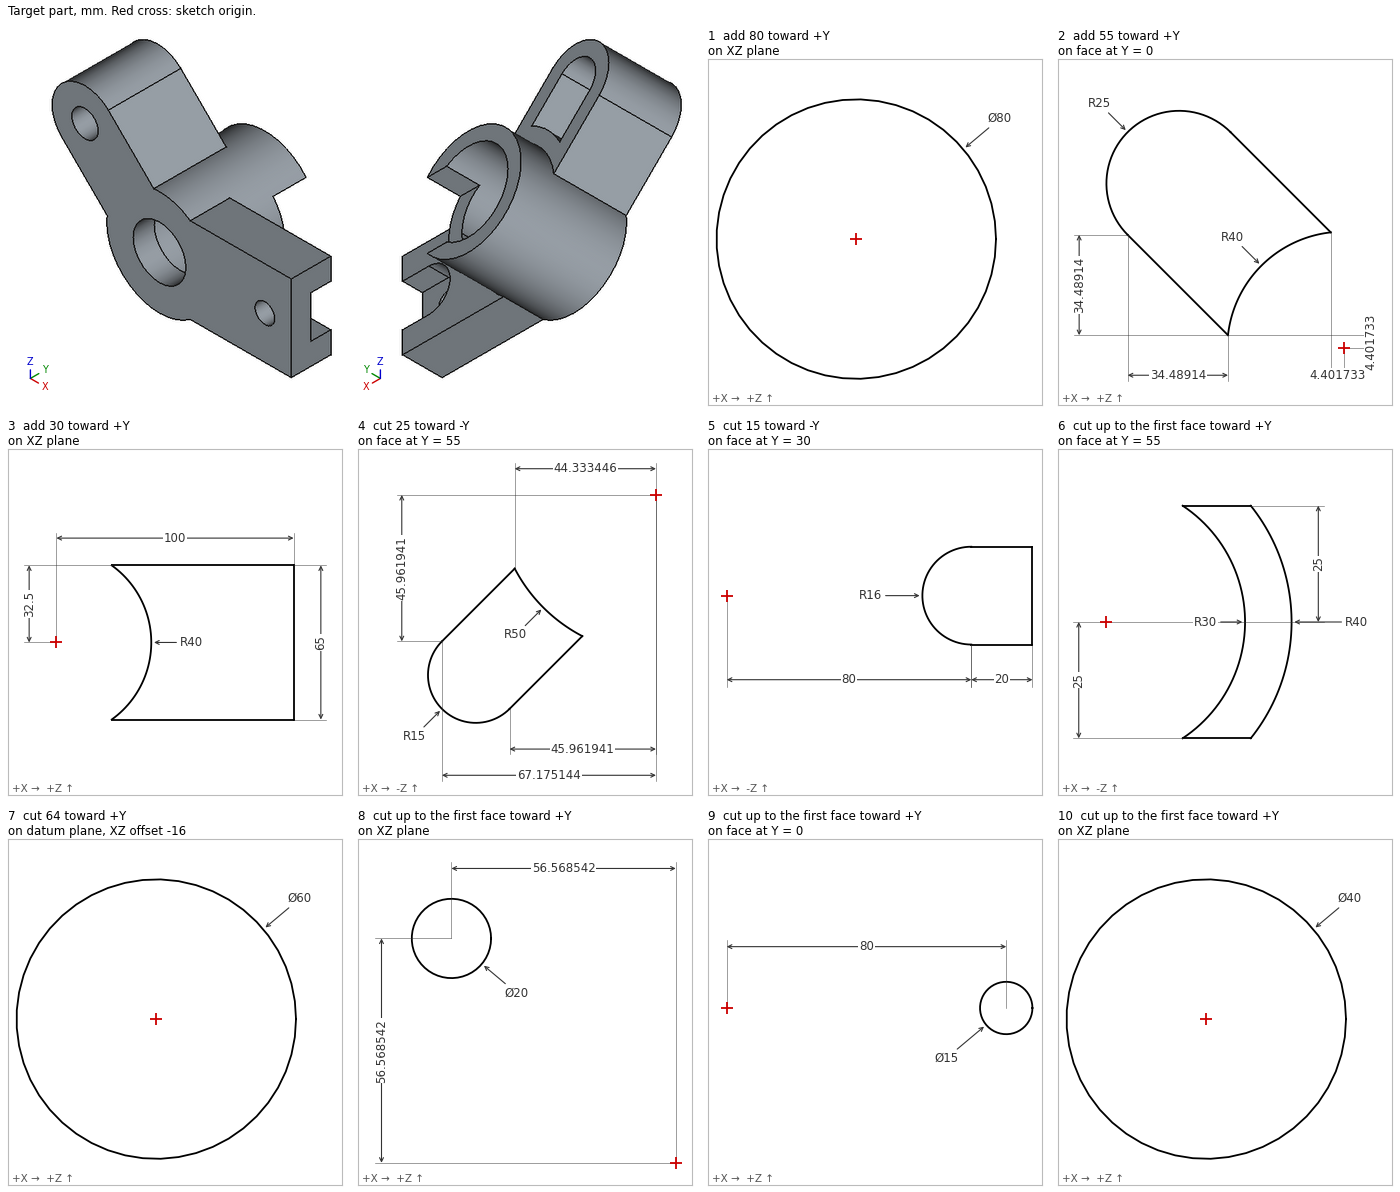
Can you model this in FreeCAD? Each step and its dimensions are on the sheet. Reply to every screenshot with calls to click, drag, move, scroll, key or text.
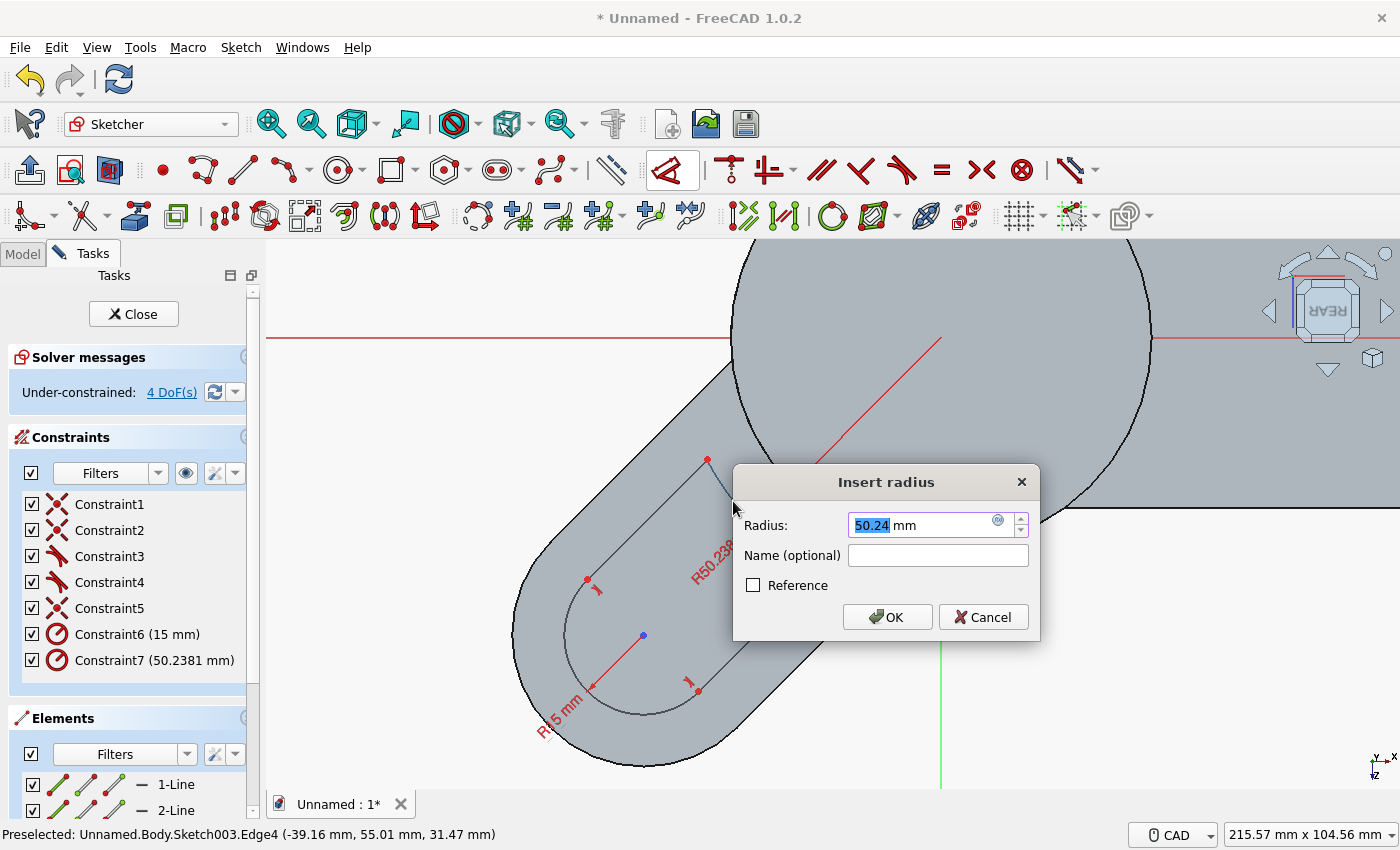
text(50)
key(Return)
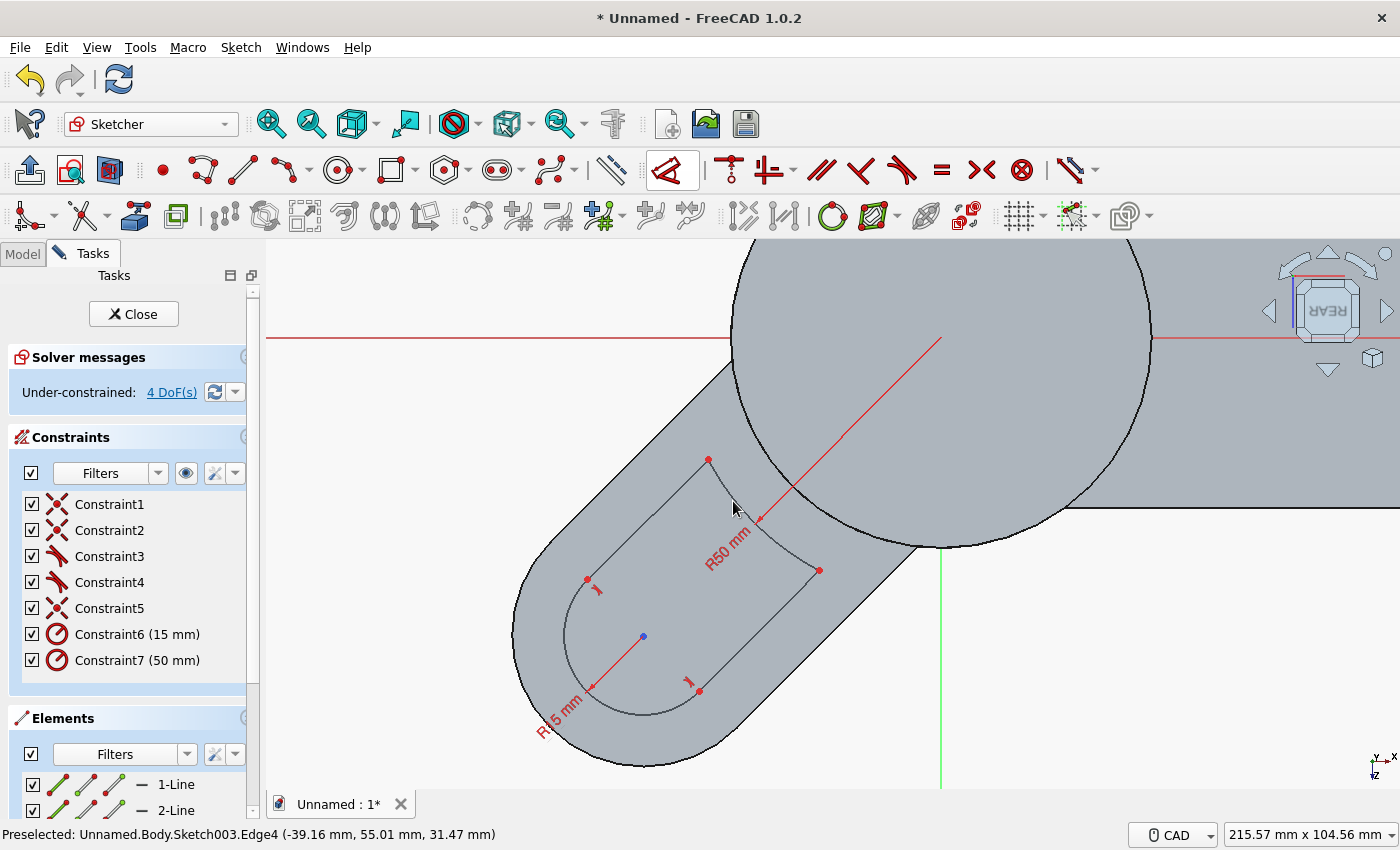
click(708, 460)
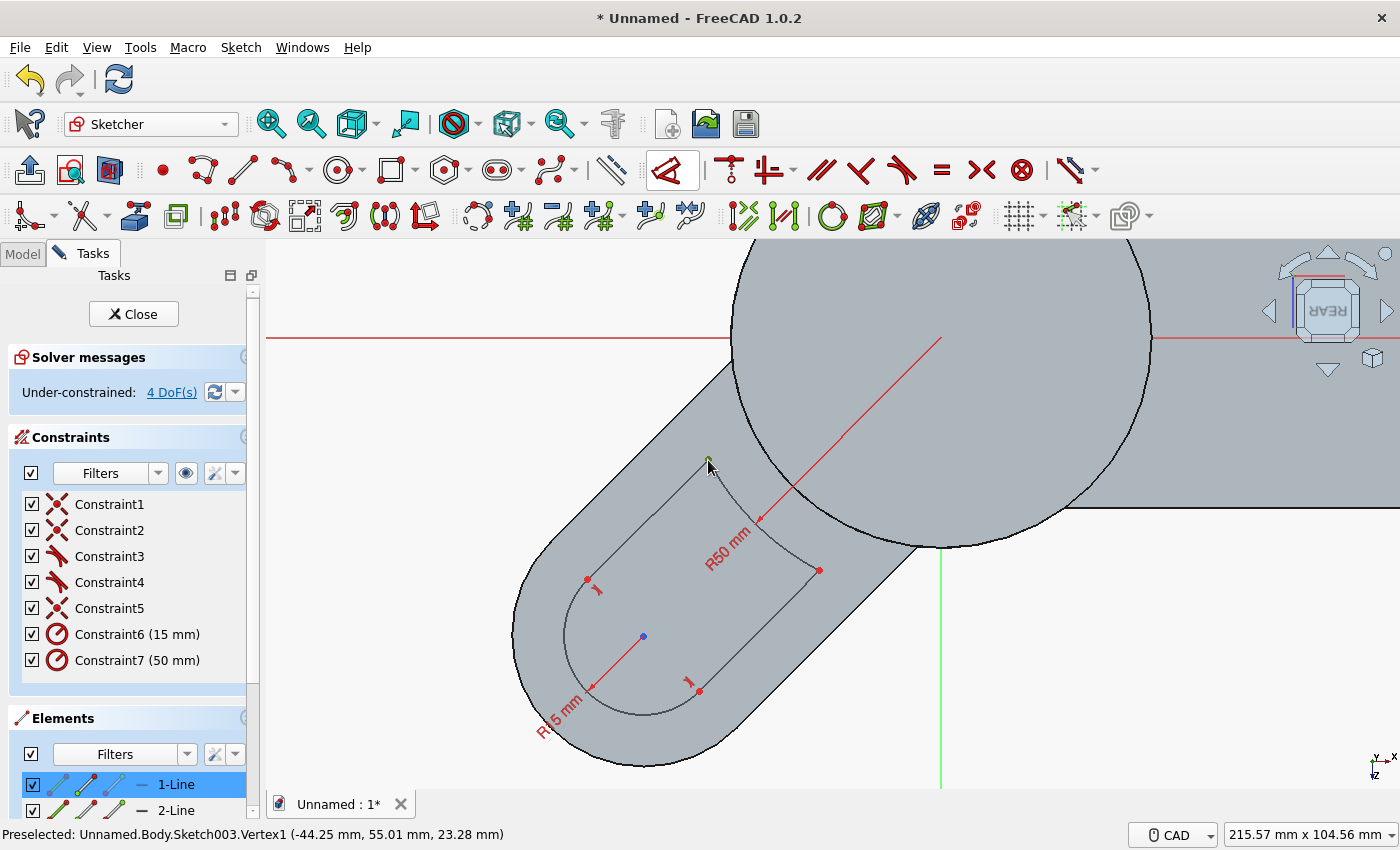
click(694, 170)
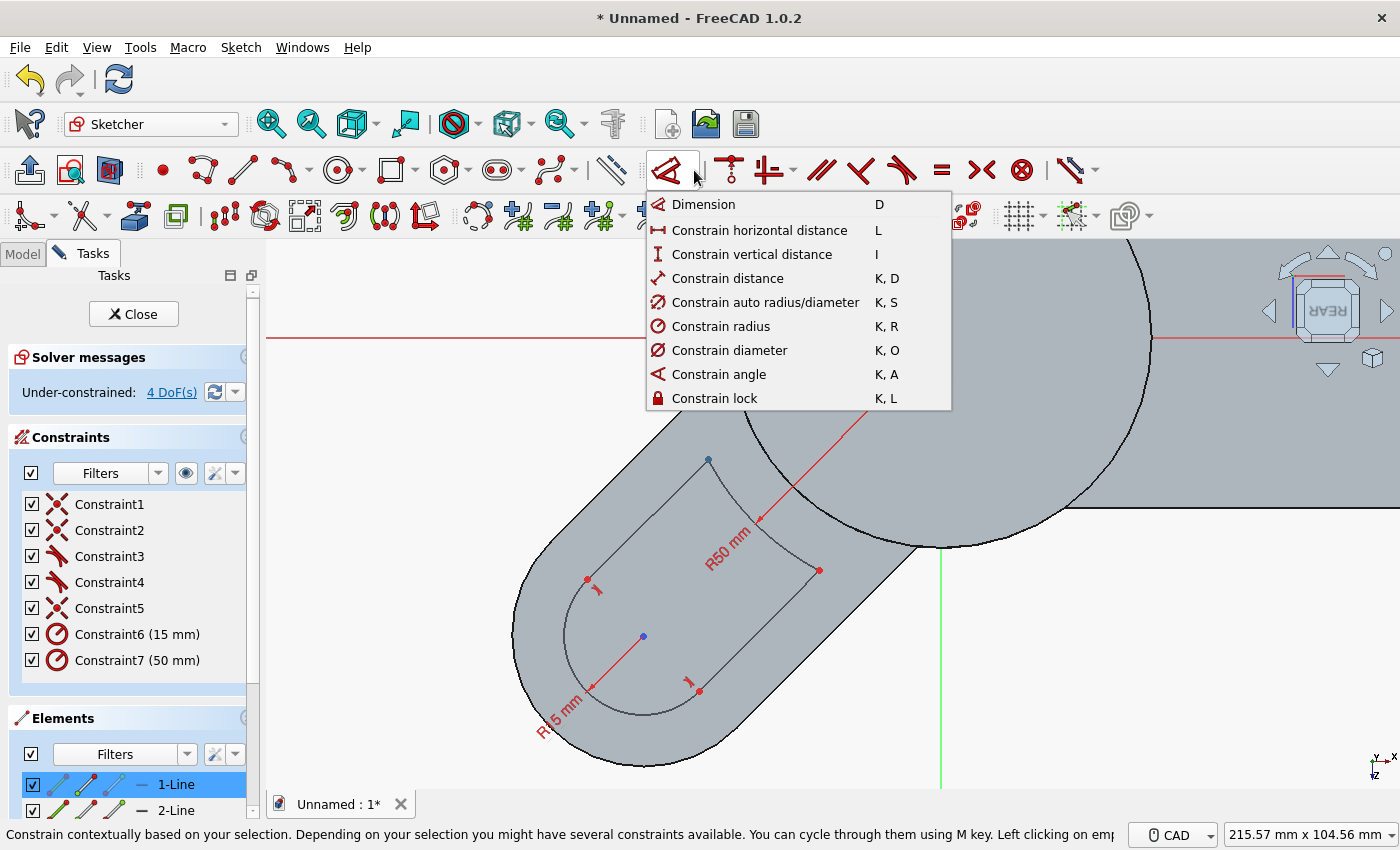
click(799, 230)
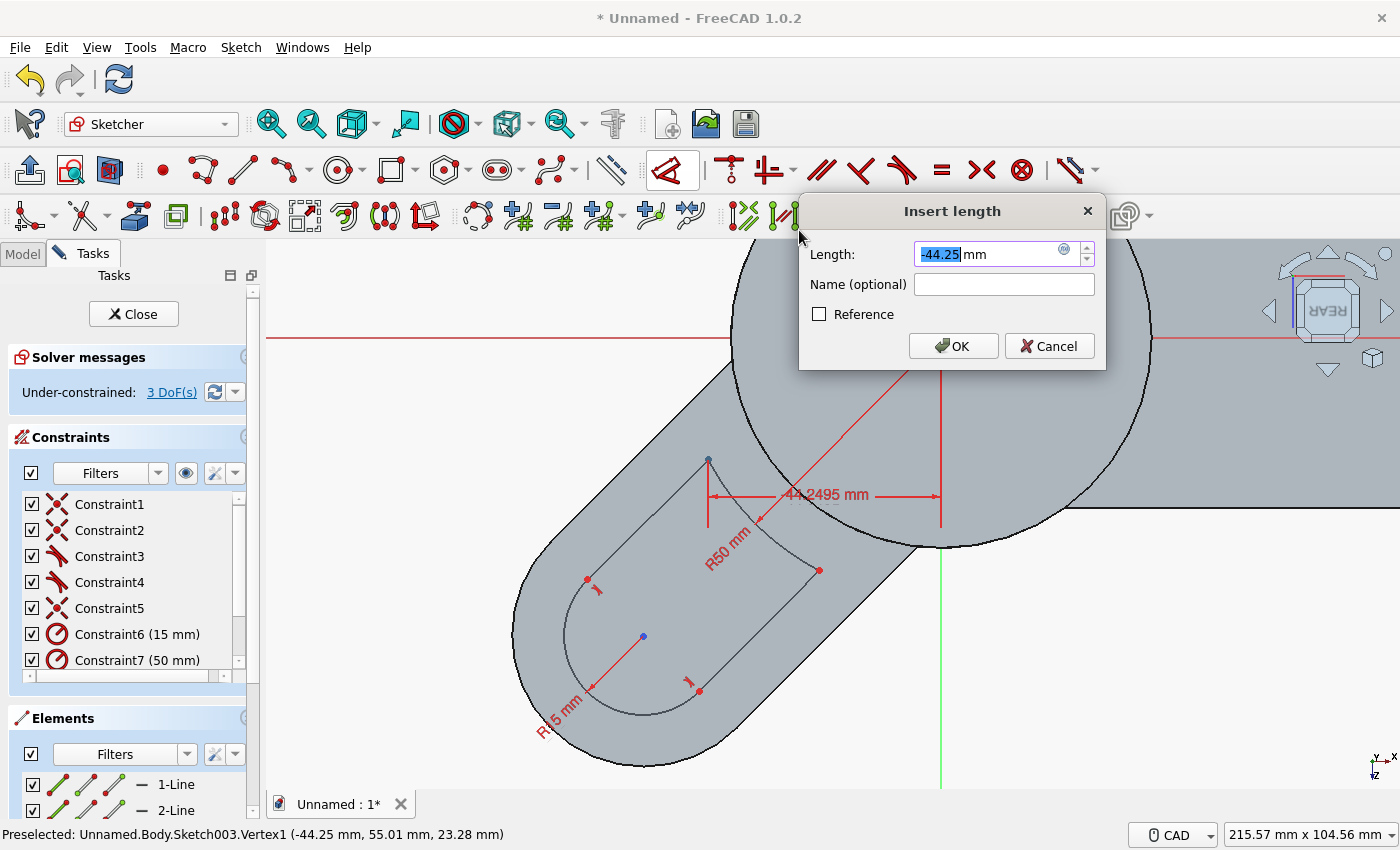
text(-44.333446)
key(Return)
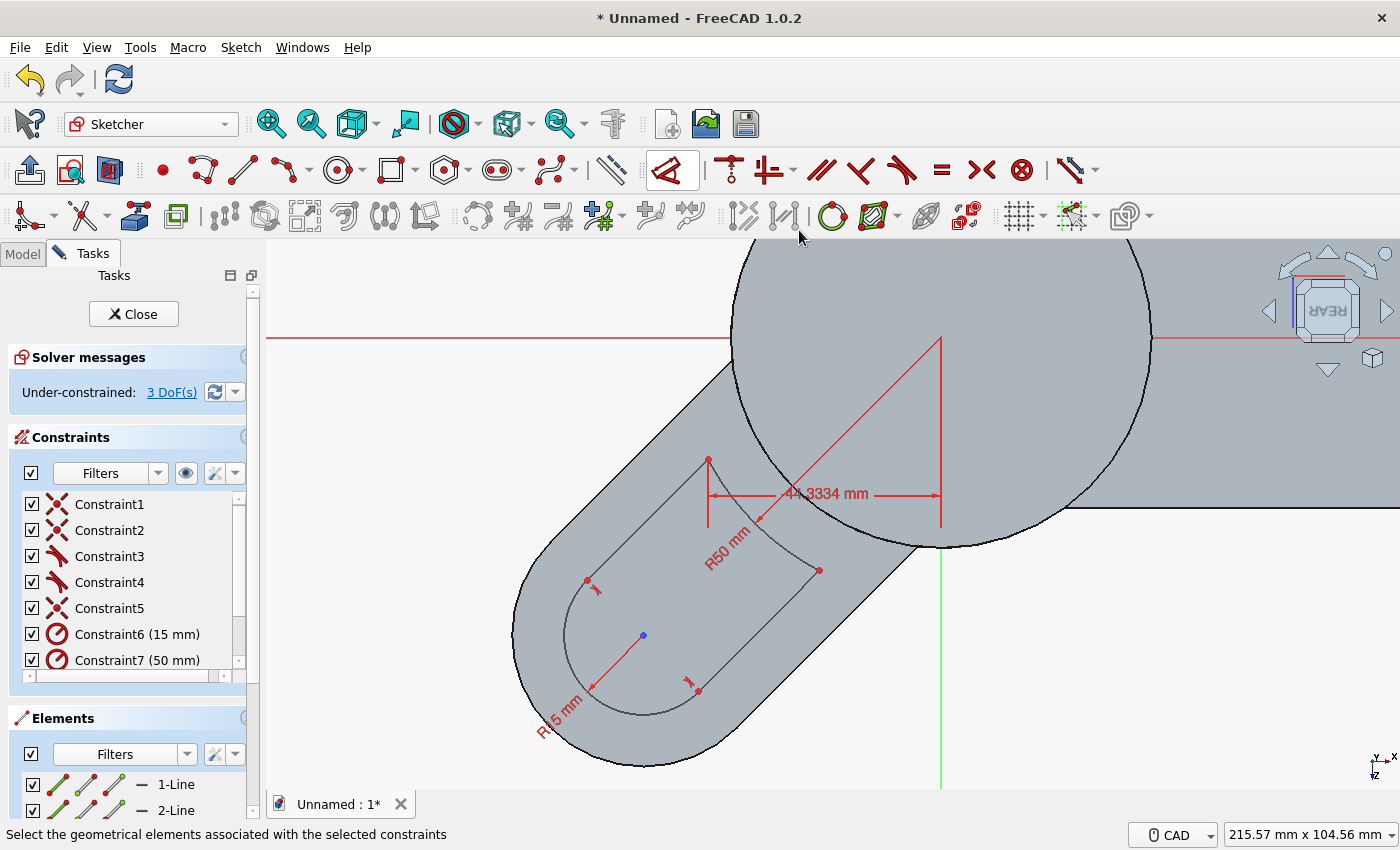
click(587, 580)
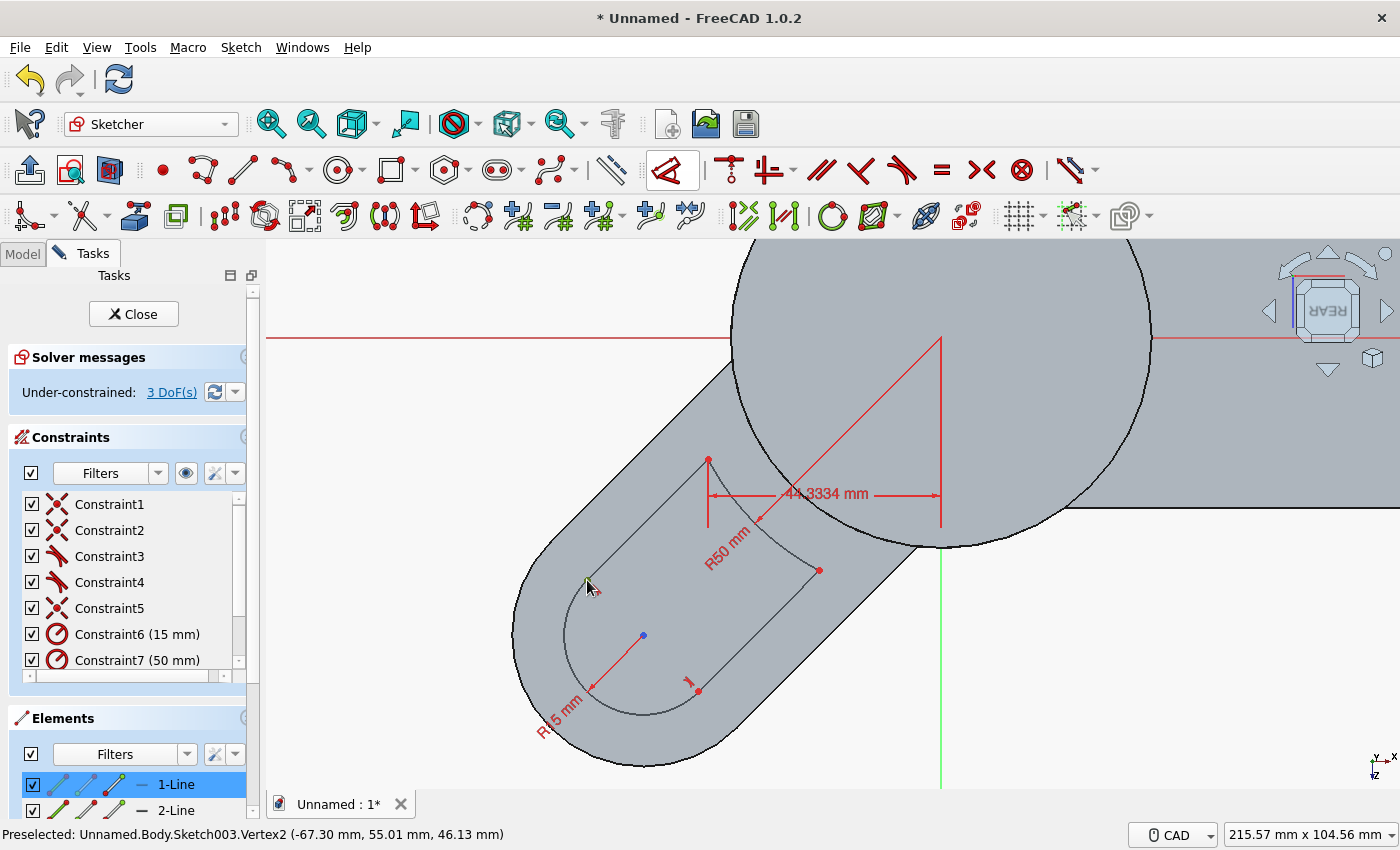
key(l)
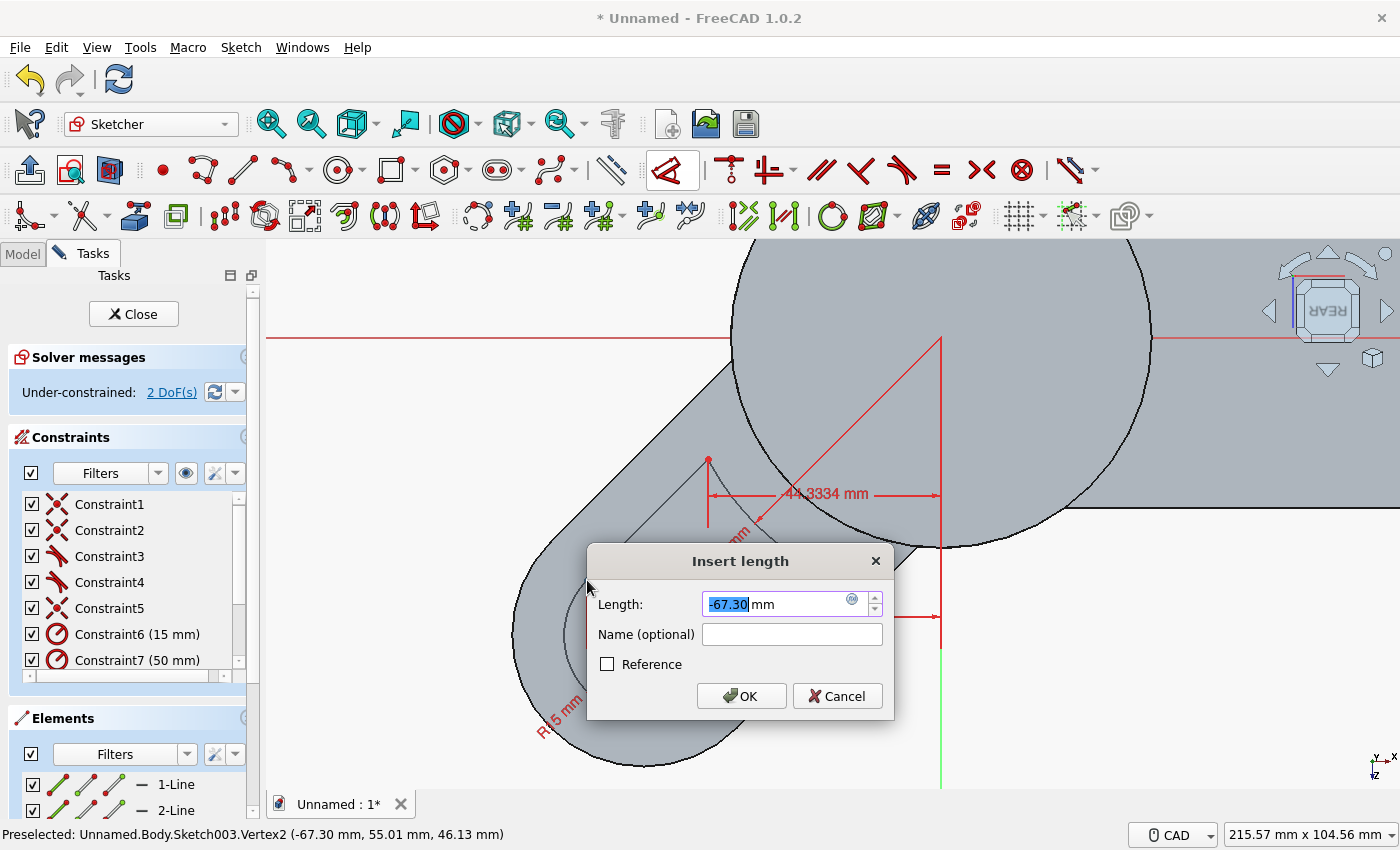
text(-67.175144)
key(Return)